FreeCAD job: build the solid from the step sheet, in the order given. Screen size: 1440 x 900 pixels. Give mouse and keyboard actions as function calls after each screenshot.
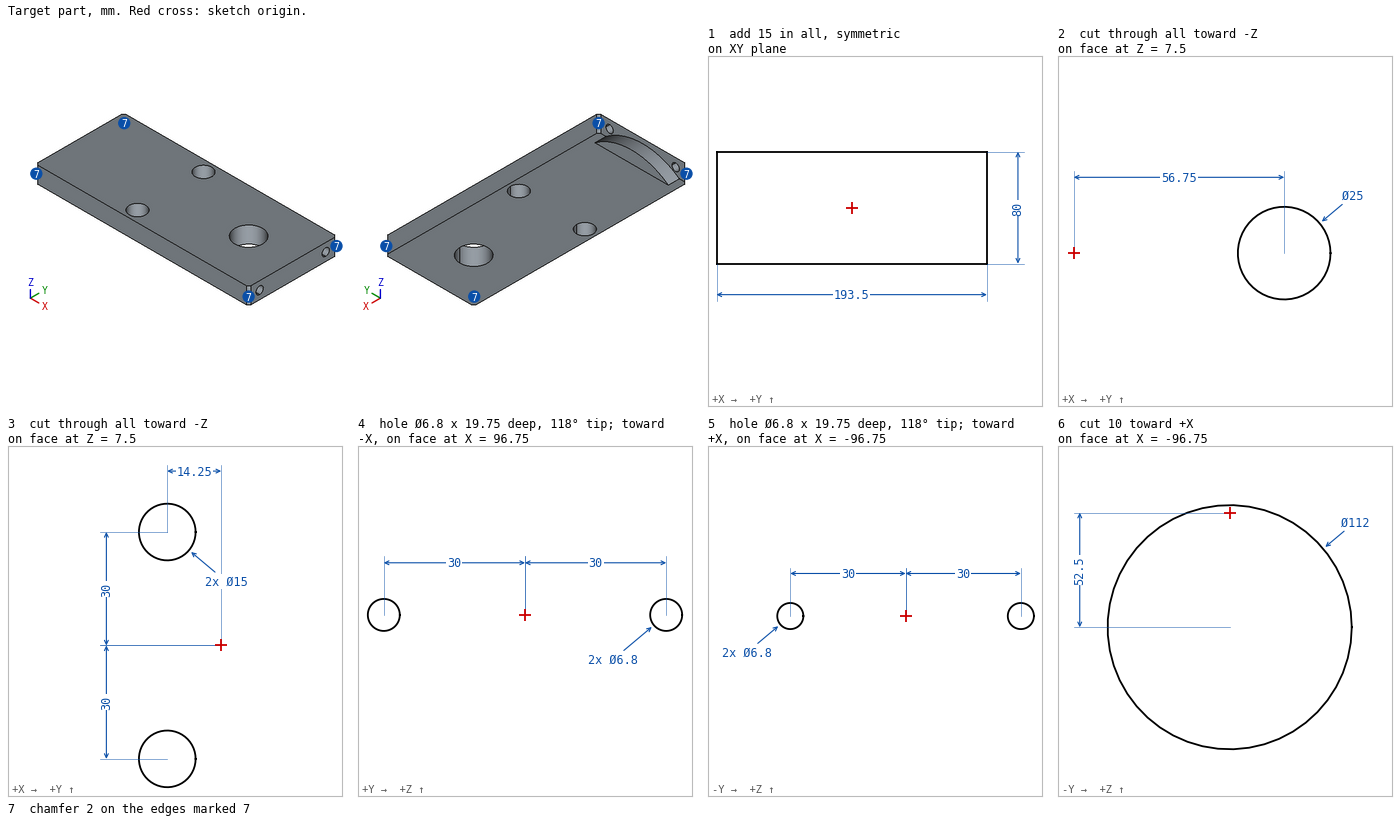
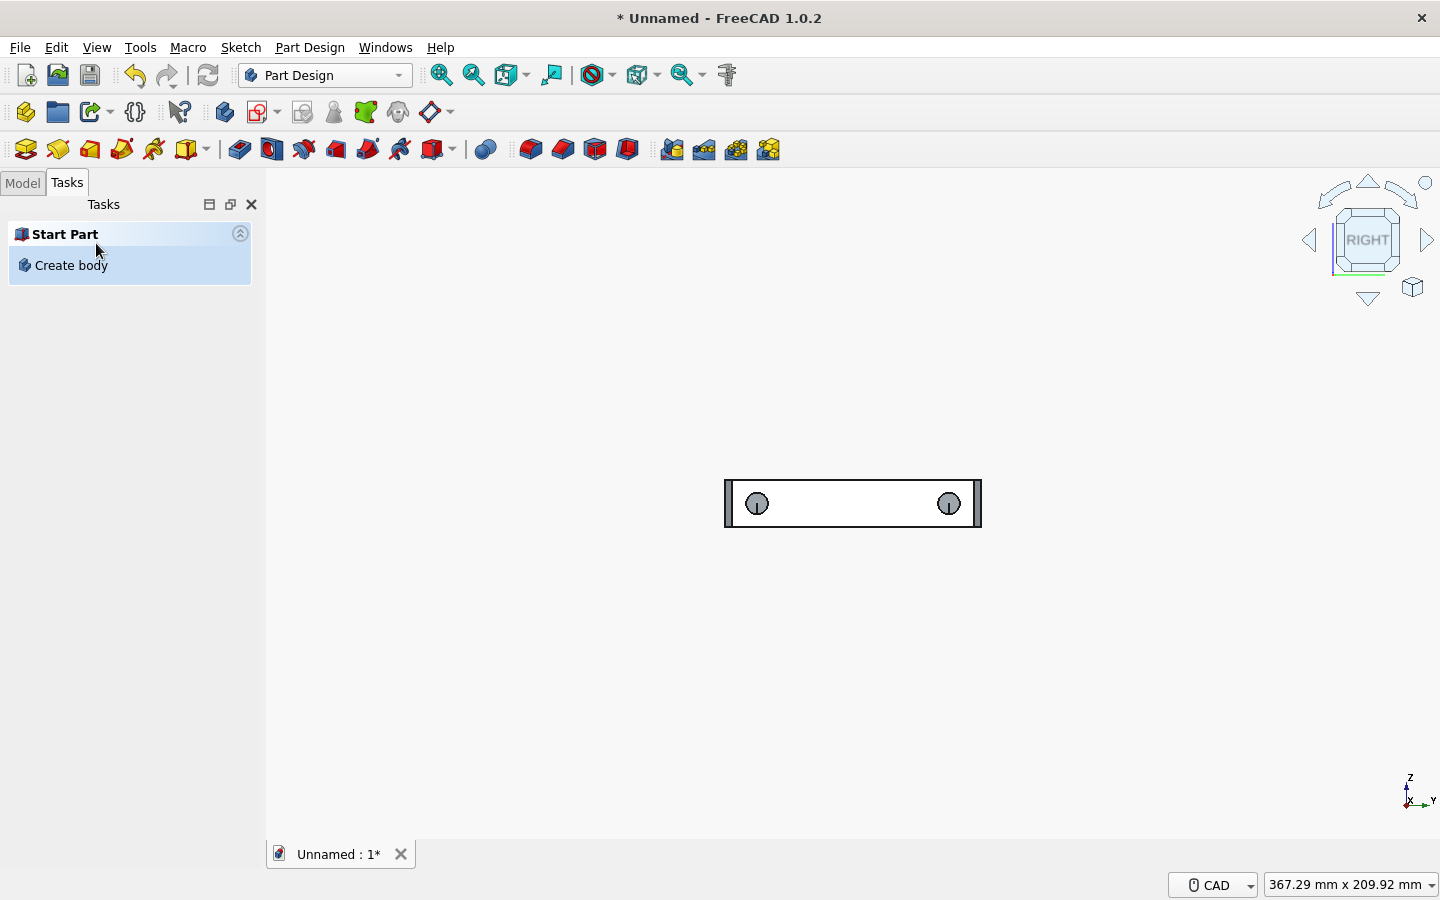
key(0)